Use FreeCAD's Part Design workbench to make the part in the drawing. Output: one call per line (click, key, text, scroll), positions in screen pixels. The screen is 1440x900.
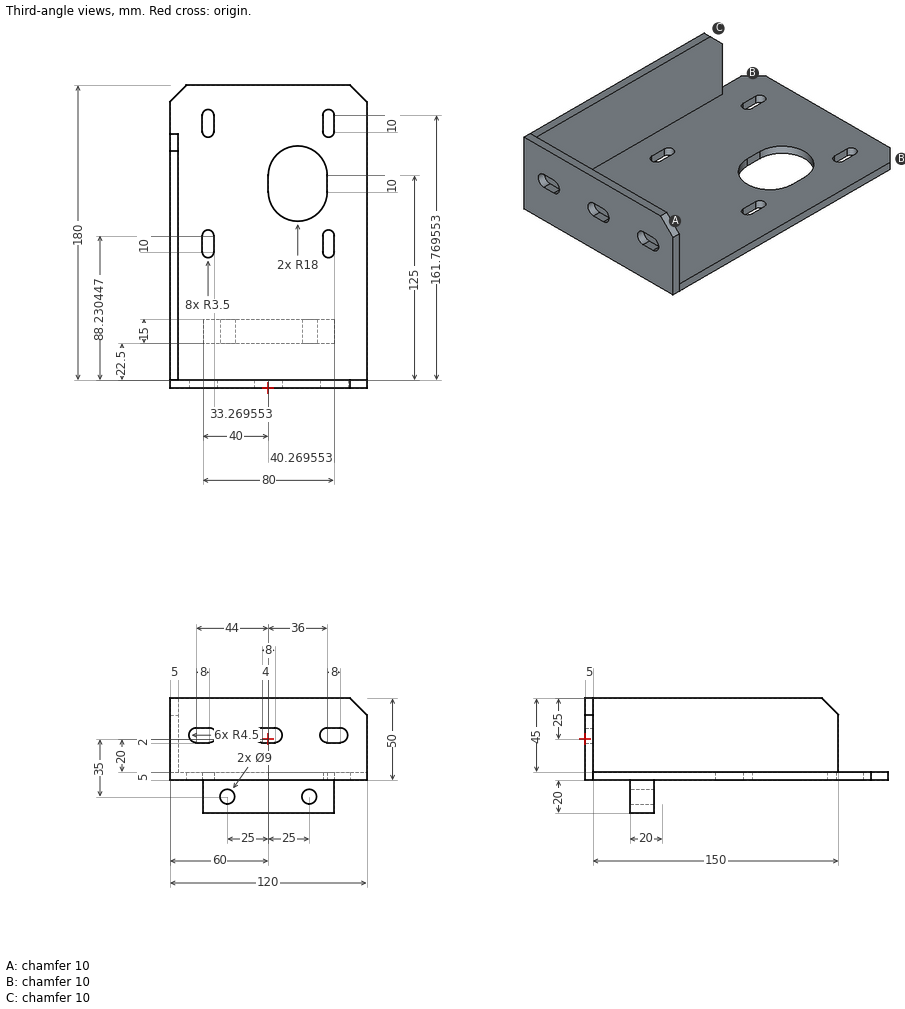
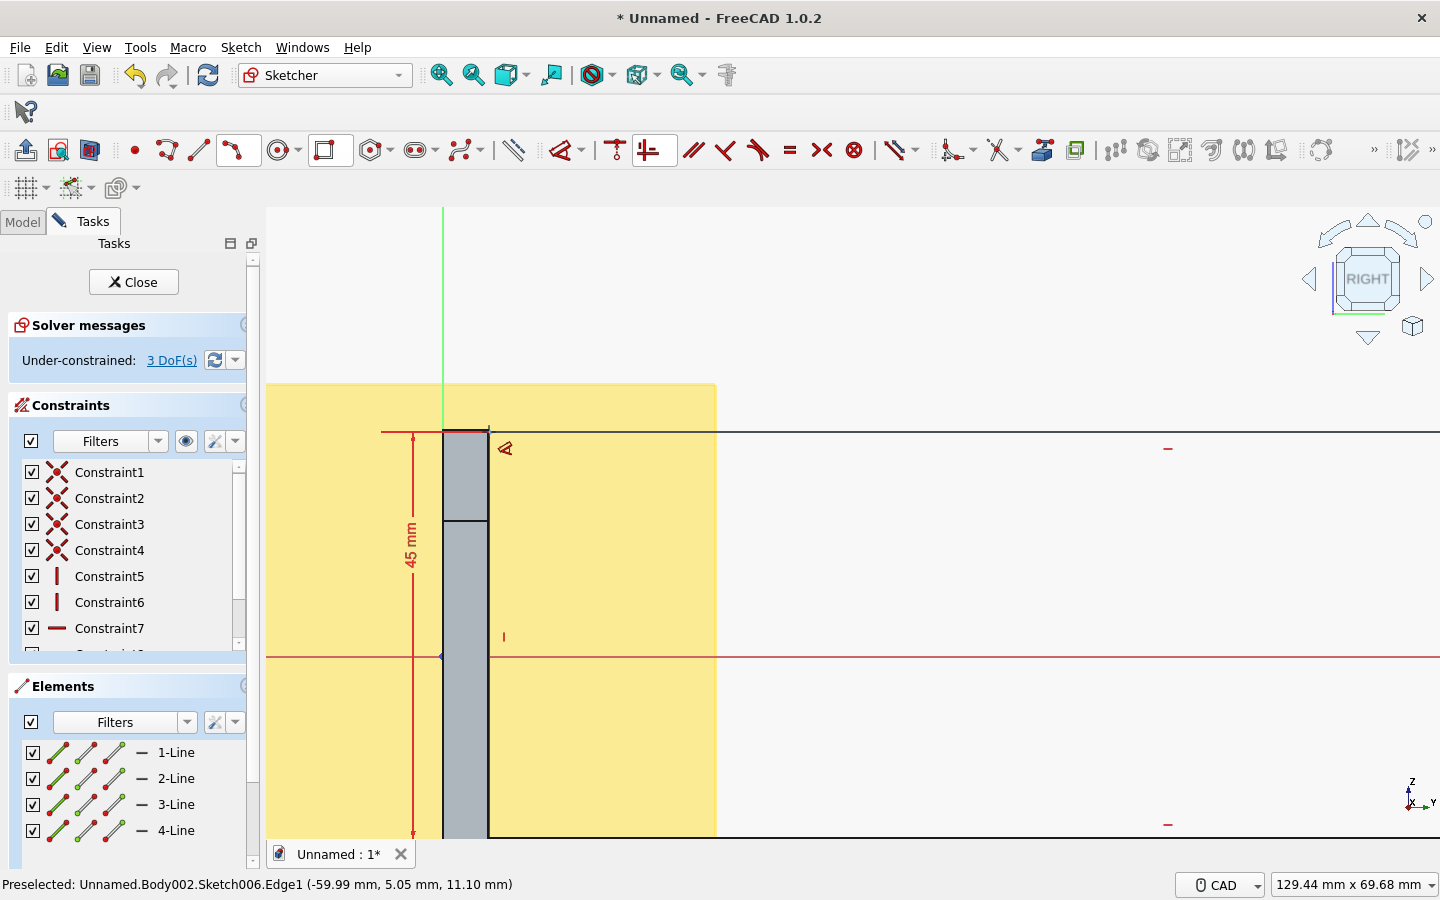
click(489, 432)
click(466, 398)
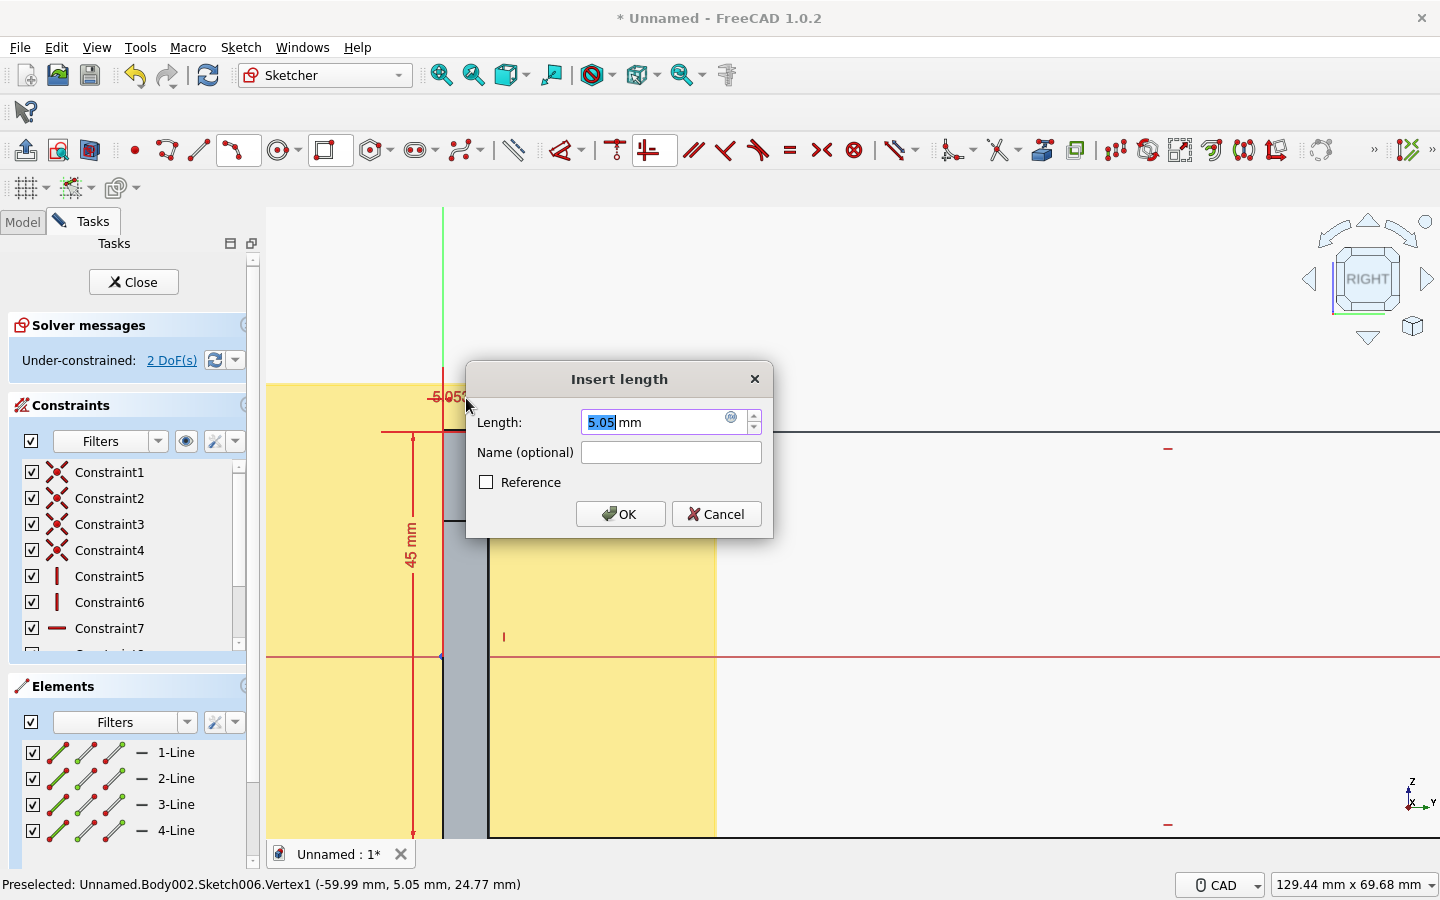
text(5)
key(Return)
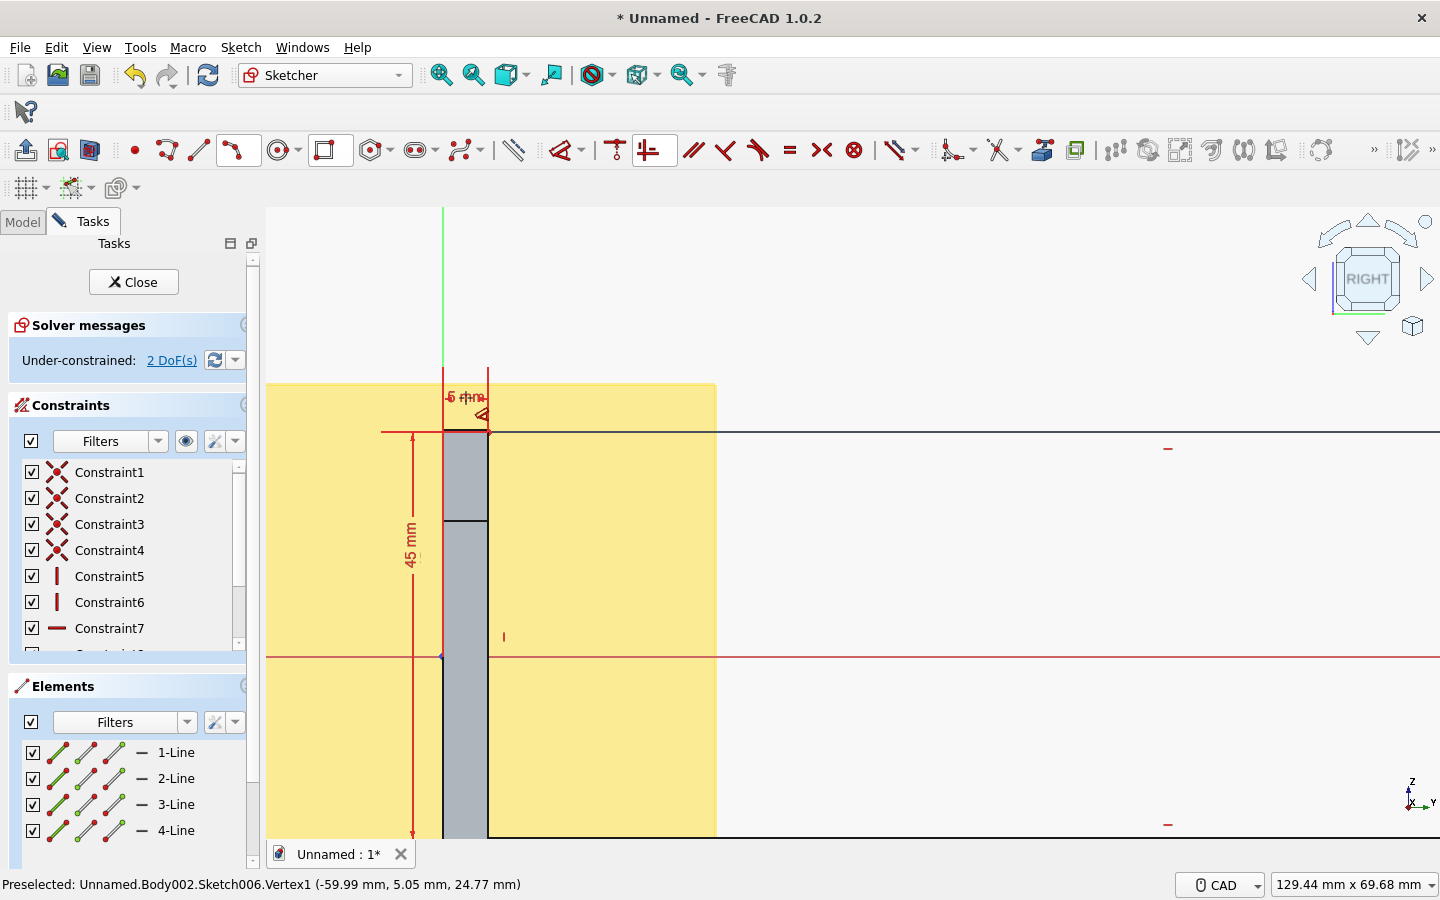
scroll(490, 432, down, 4)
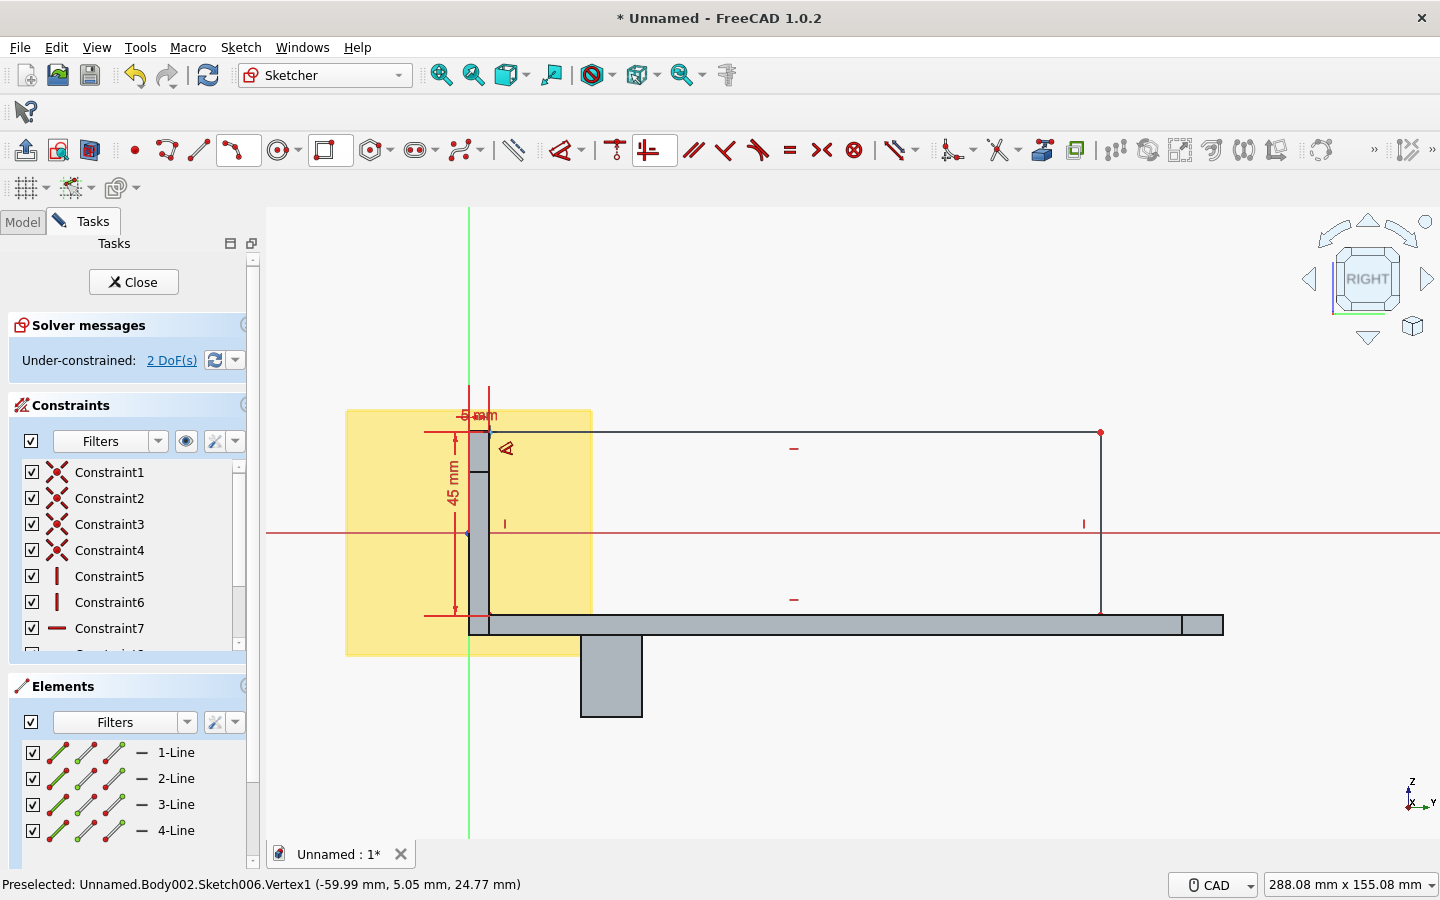
click(673, 616)
click(795, 650)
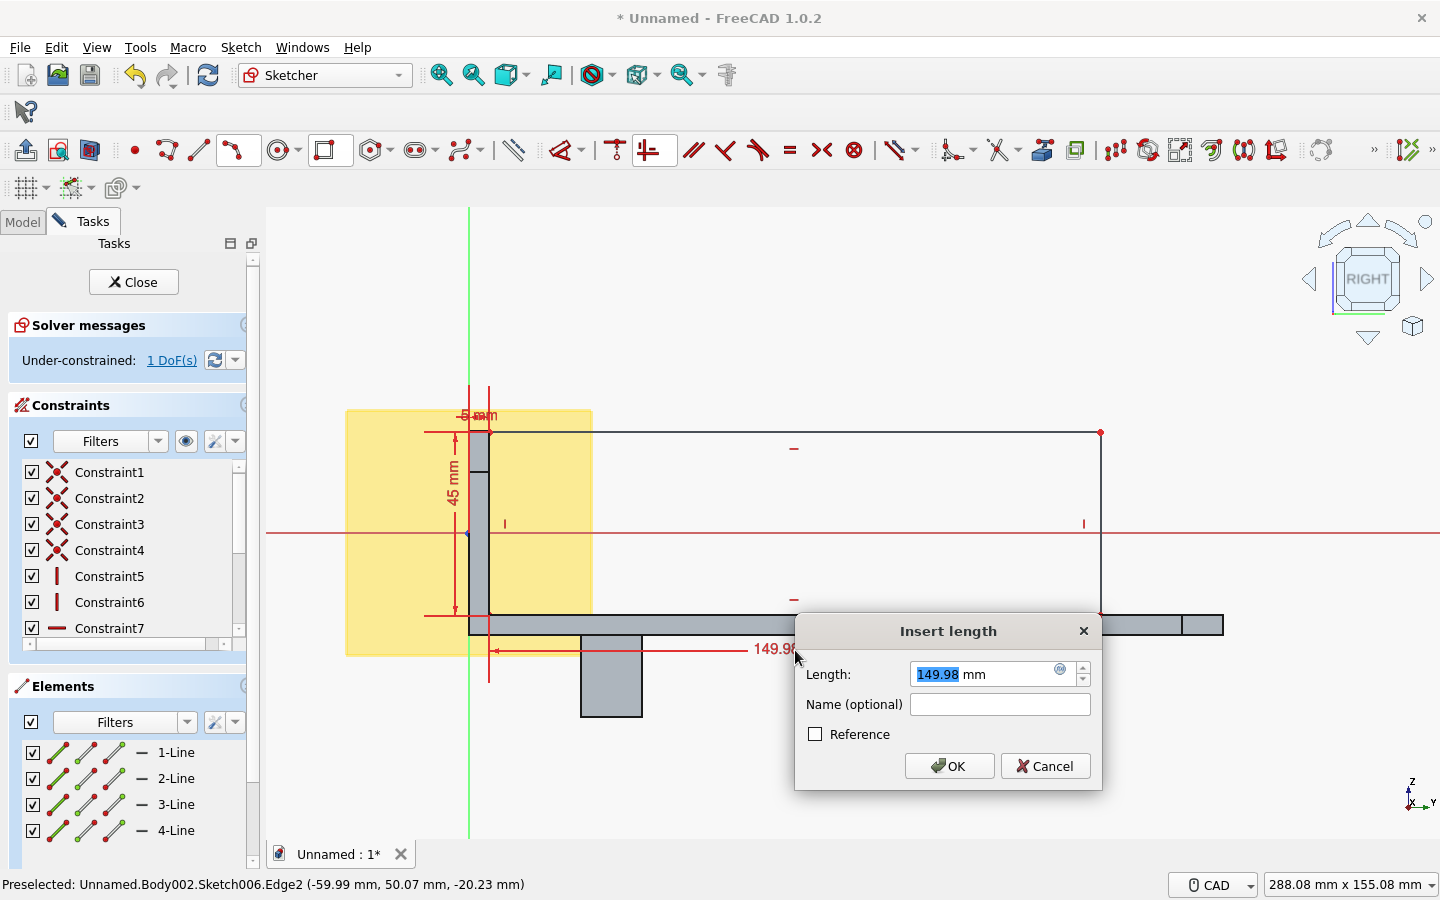
text(150)
key(Return)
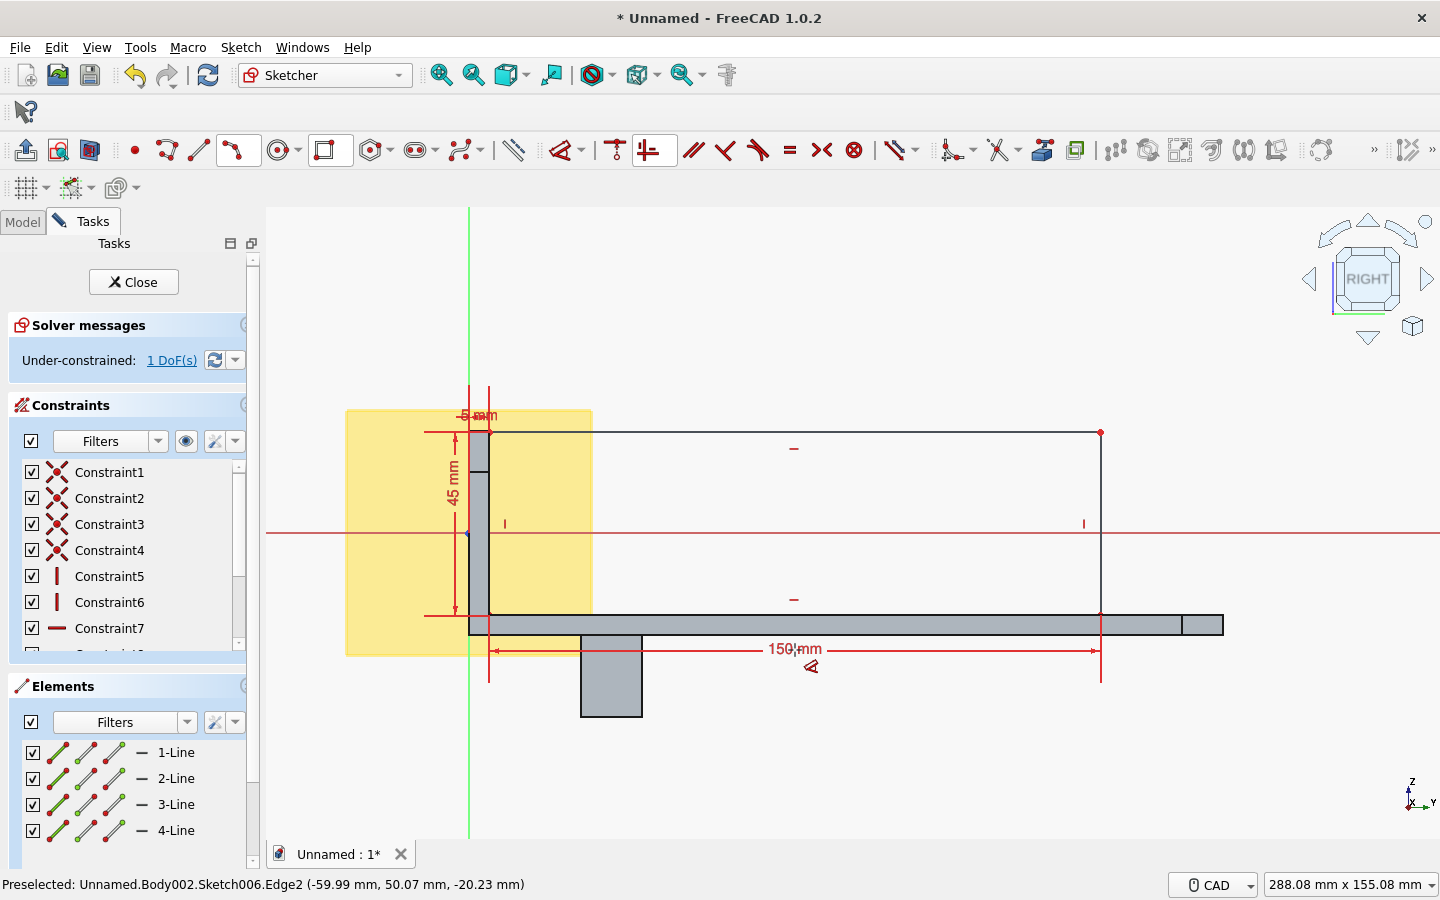
click(489, 432)
click(435, 460)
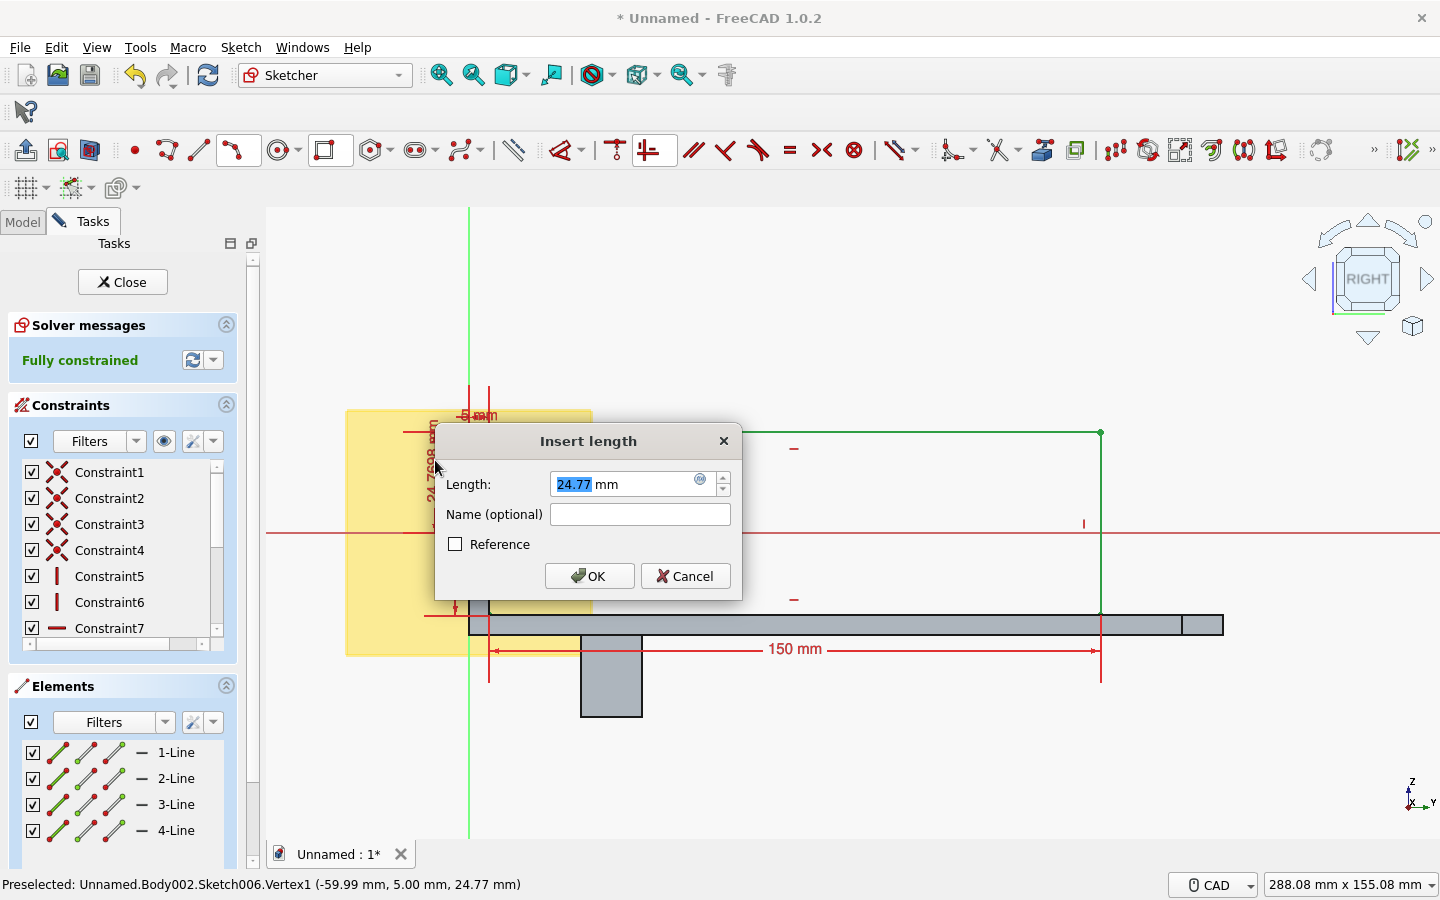
text(25)
key(Return)
key(Escape)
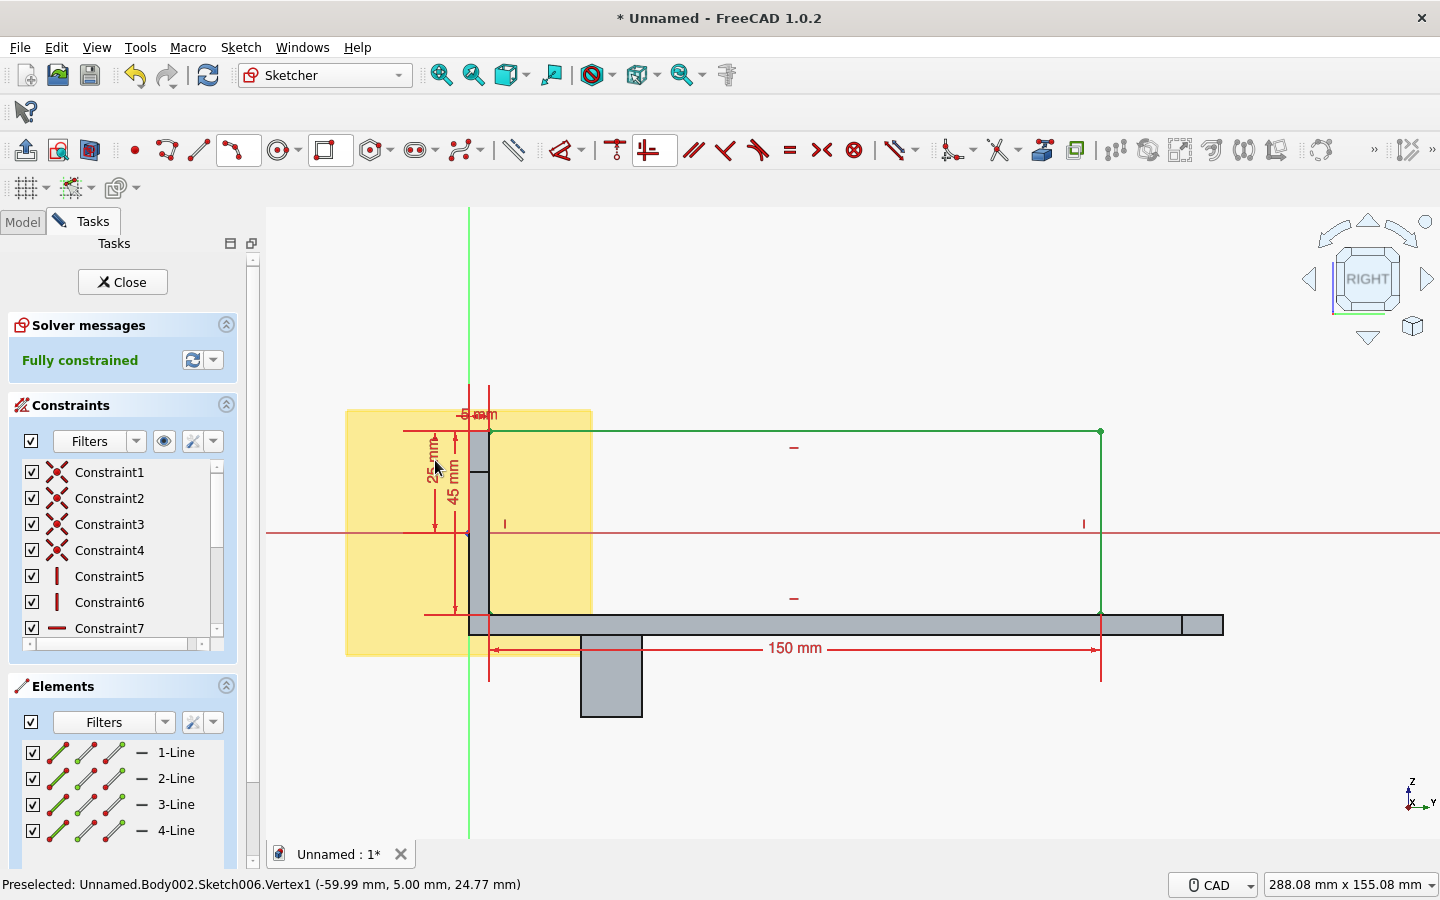
click(123, 282)